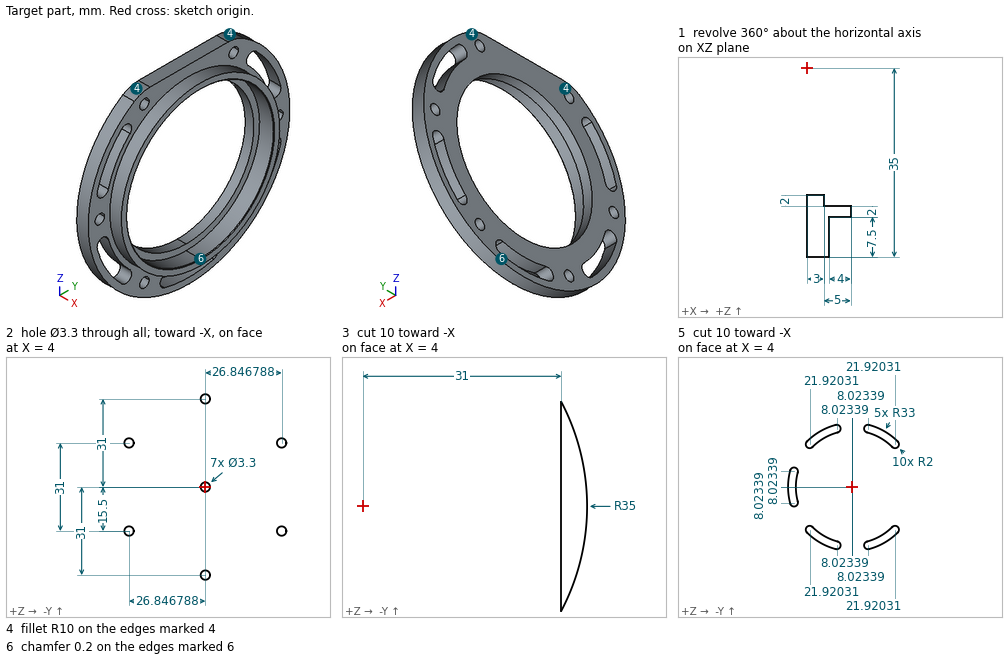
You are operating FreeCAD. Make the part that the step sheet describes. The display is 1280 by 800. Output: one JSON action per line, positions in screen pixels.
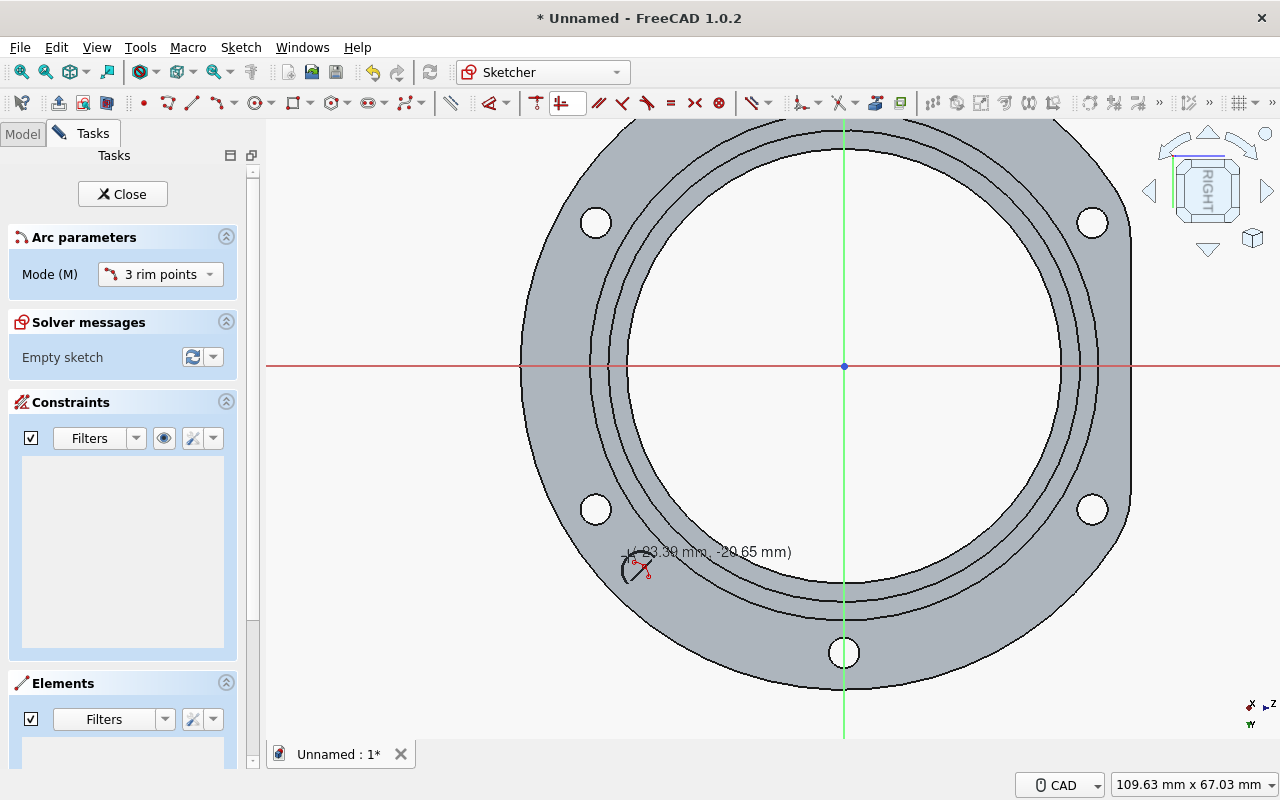
{"action": "left_click", "coordinate": [628, 556]}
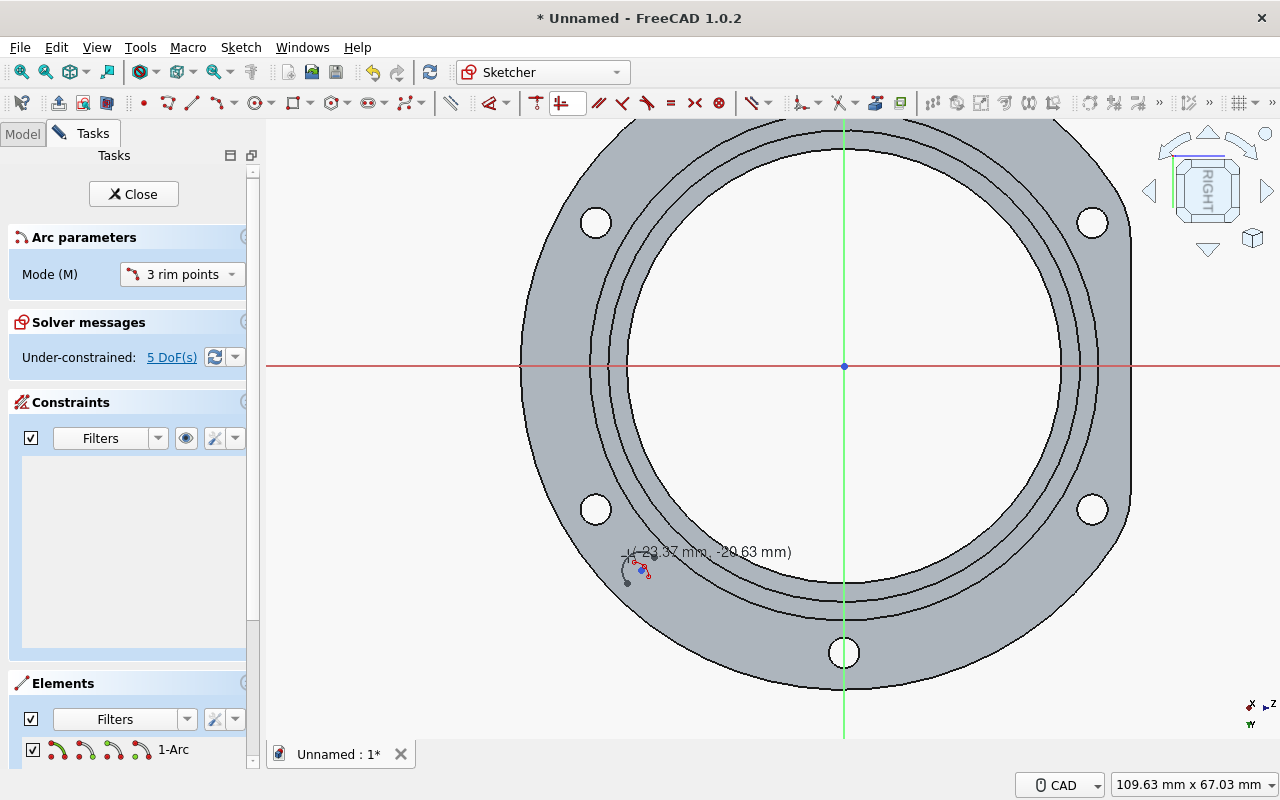
{"action": "left_click", "coordinate": [628, 584]}
{"action": "left_click", "coordinate": [765, 661]}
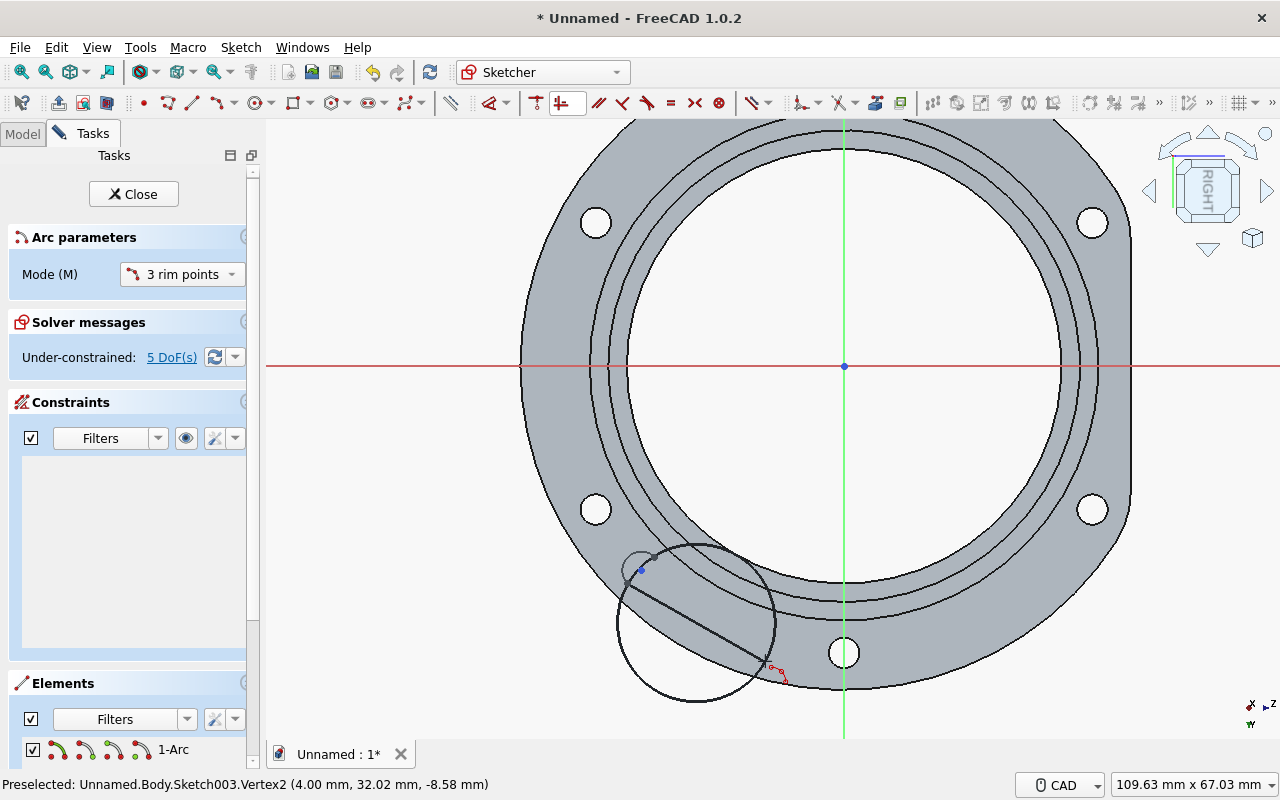
{"action": "scroll", "coordinate": [692, 631], "scroll_direction": "up", "scroll_amount": 3}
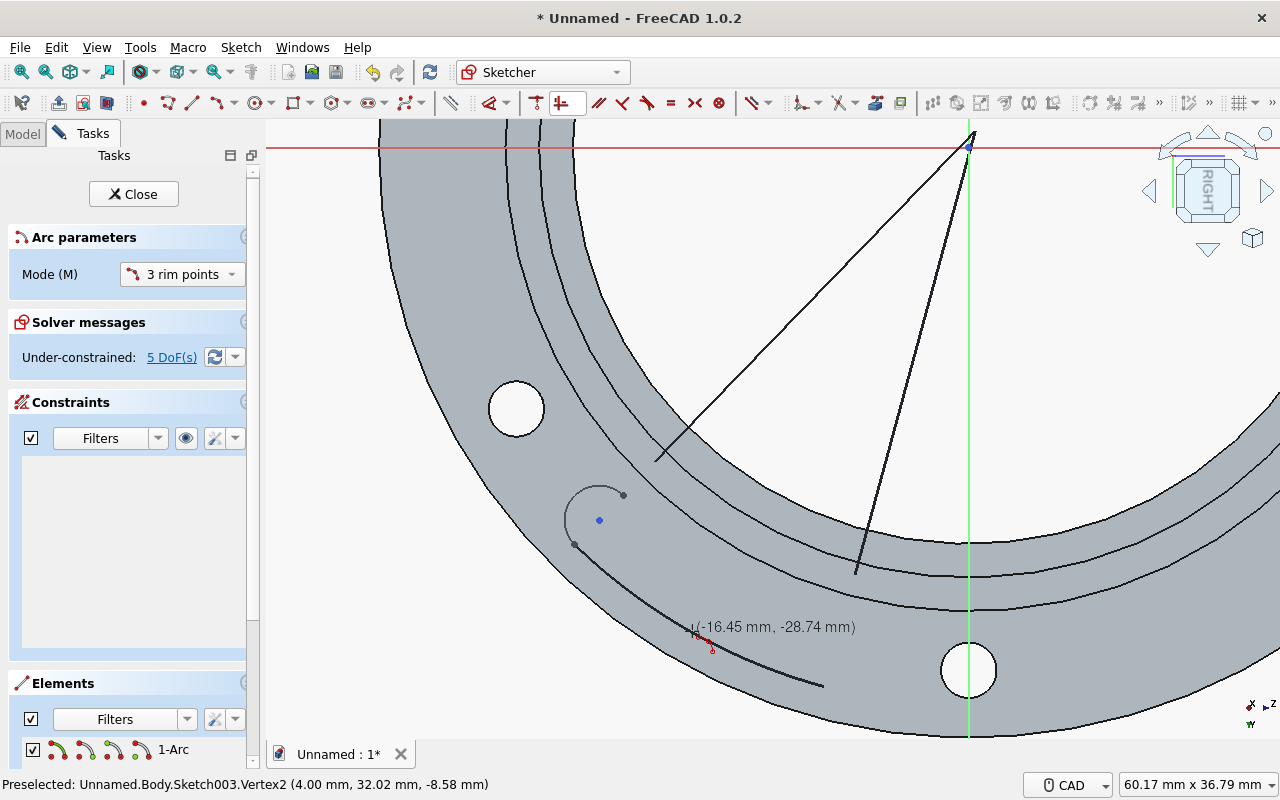
{"action": "left_click", "coordinate": [691, 629]}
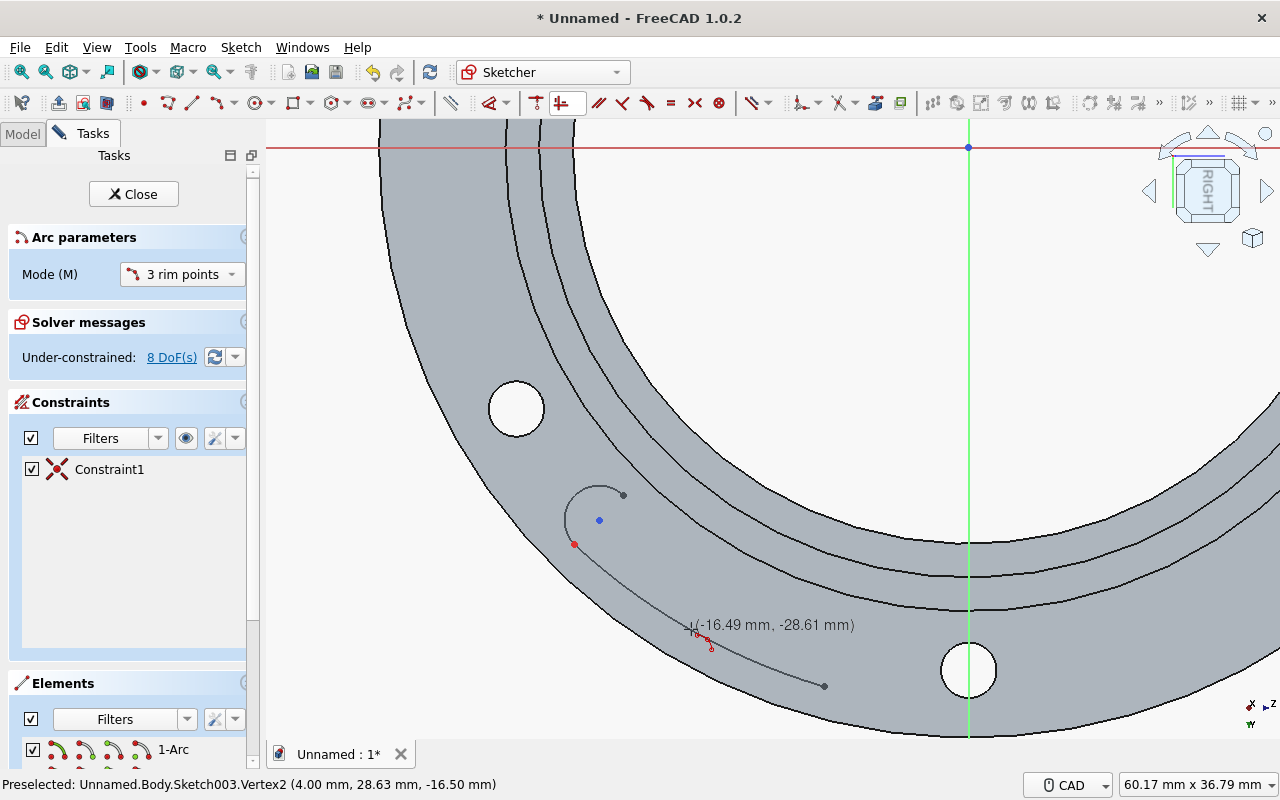
{"action": "left_click", "coordinate": [825, 687]}
{"action": "left_click", "coordinate": [842, 620]}
{"action": "left_click", "coordinate": [866, 661]}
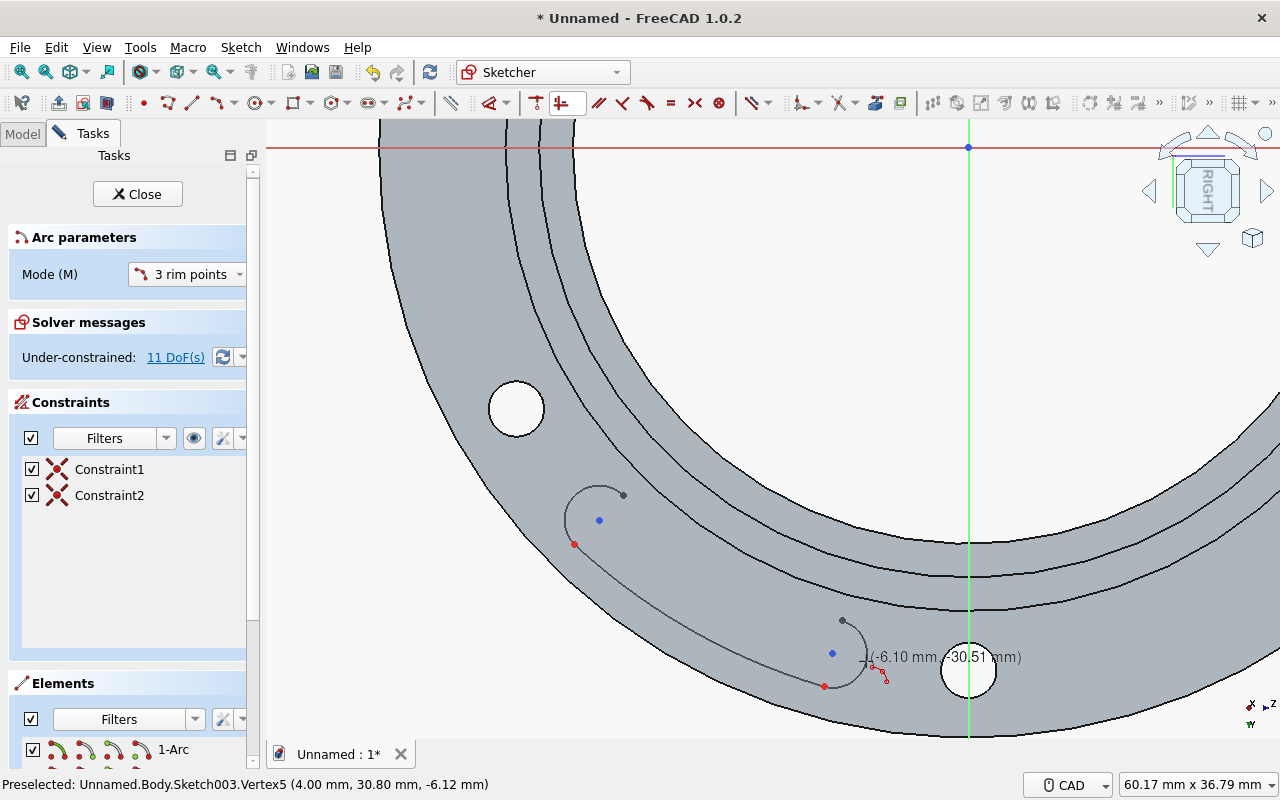
{"action": "left_click", "coordinate": [842, 621]}
{"action": "left_click", "coordinate": [624, 496]}
{"action": "left_click", "coordinate": [724, 571]}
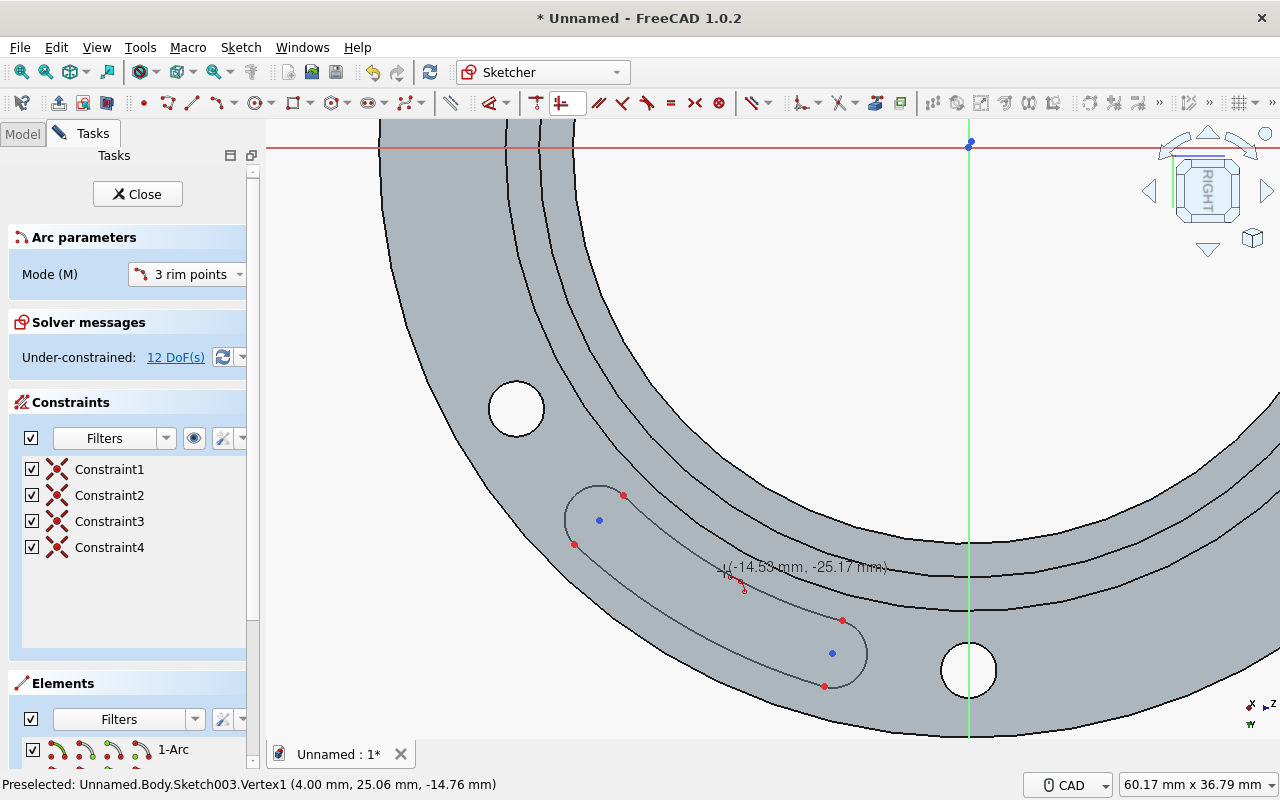
{"action": "left_click", "coordinate": [497, 274]}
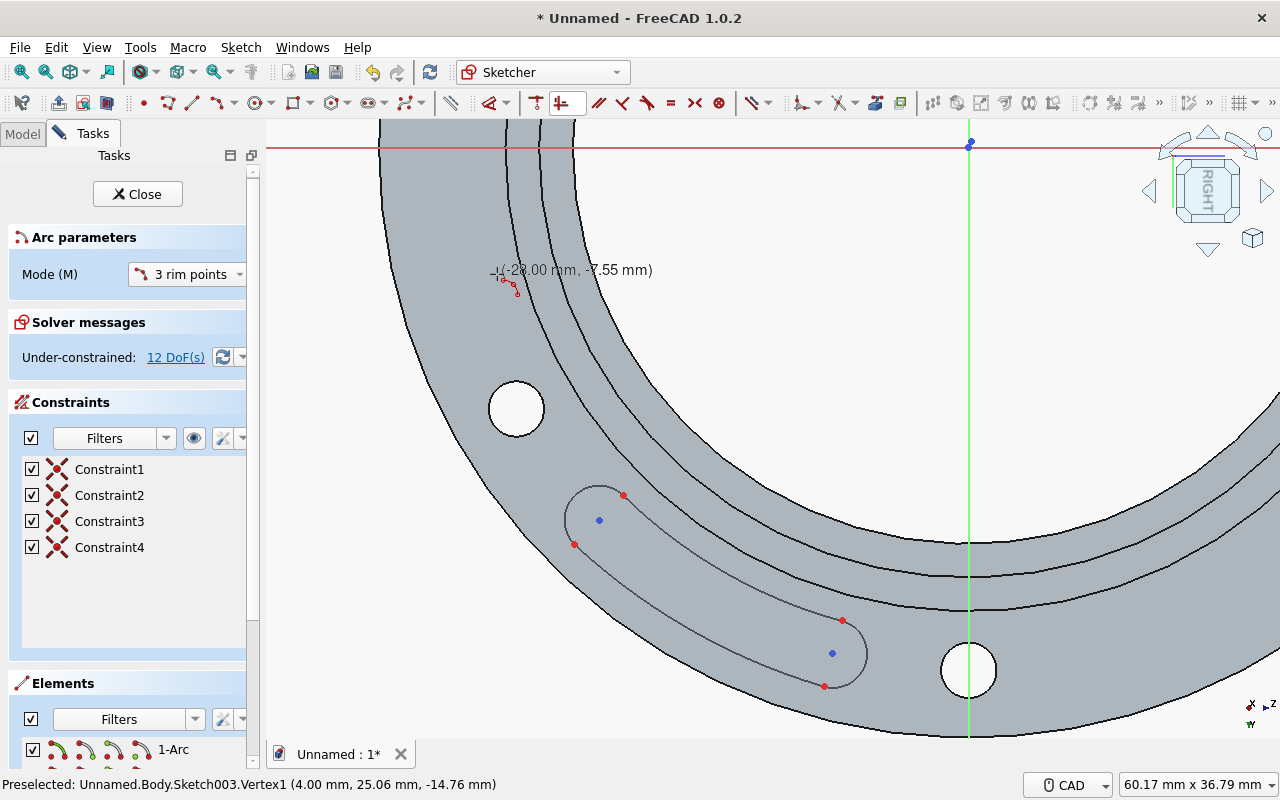
{"action": "scroll", "coordinate": [598, 593], "scroll_direction": "down", "scroll_amount": 5}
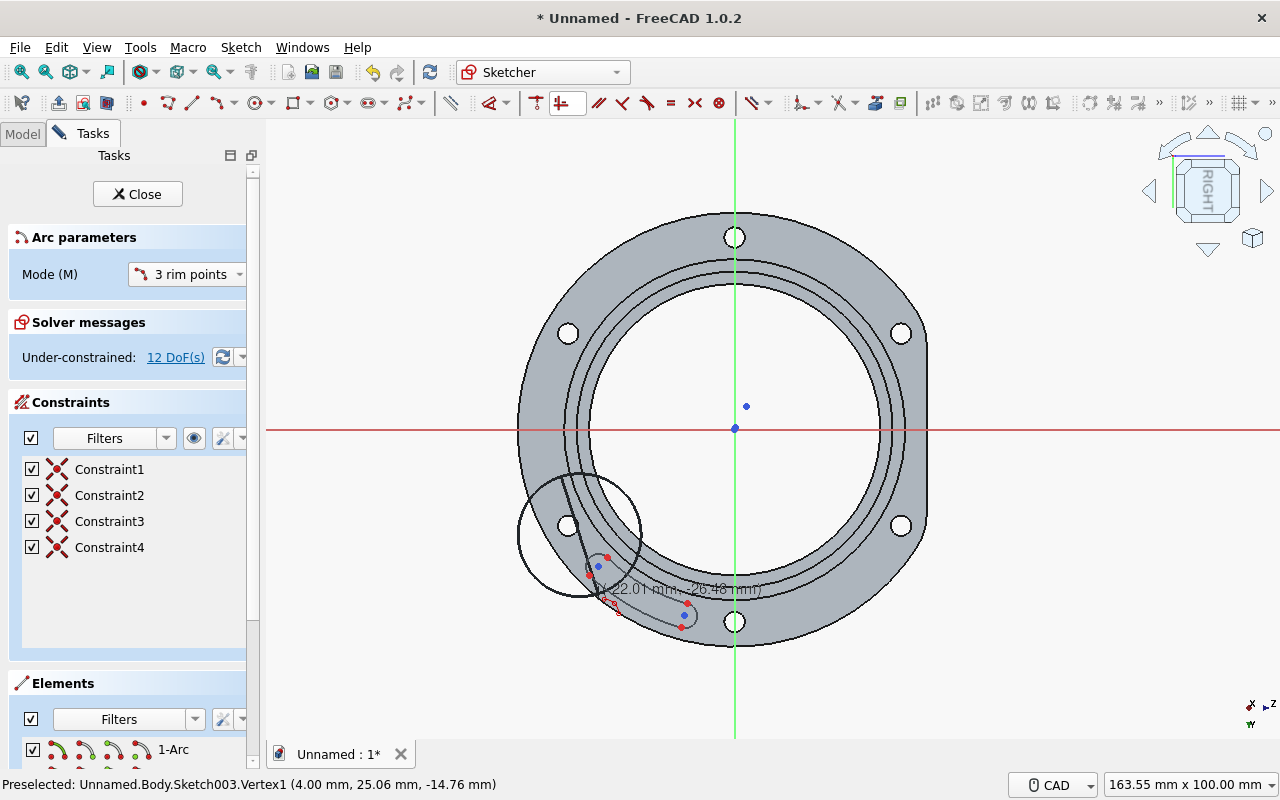
{"action": "left_click", "coordinate": [561, 383]}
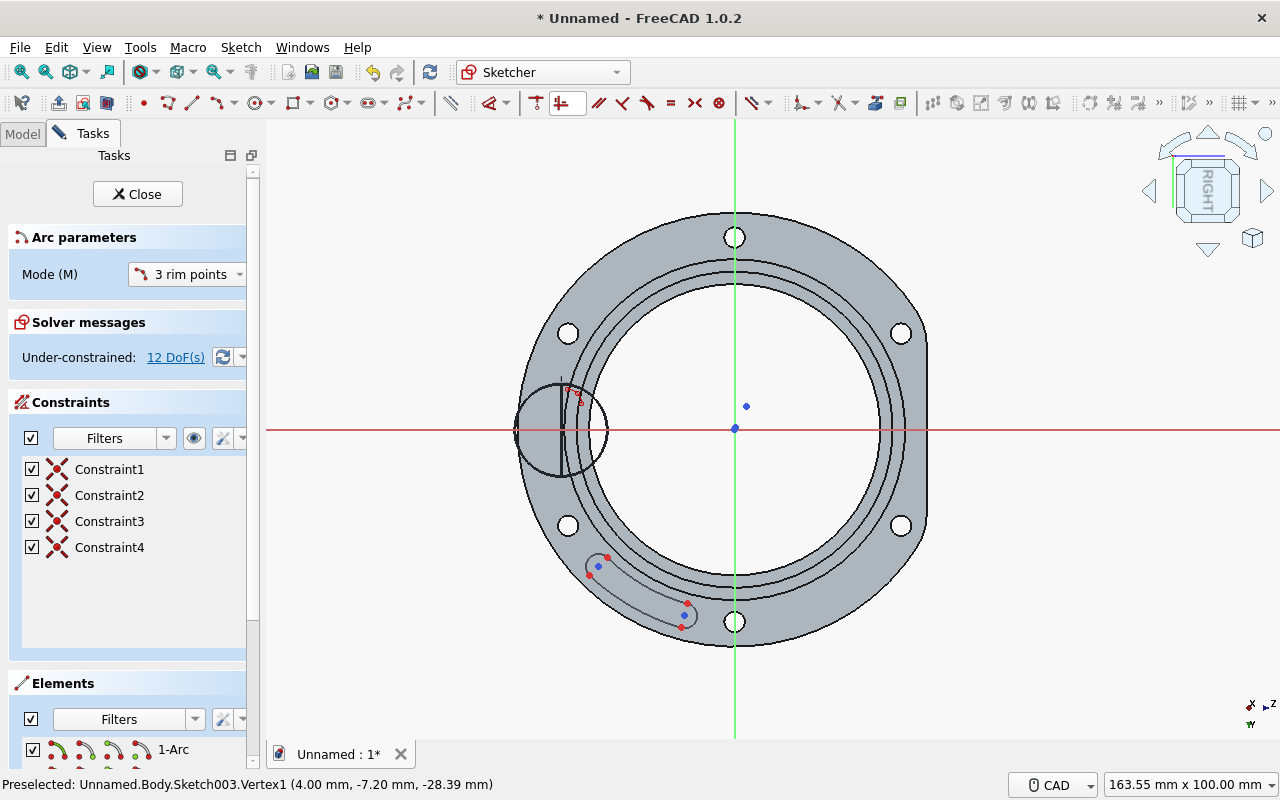
{"action": "scroll", "coordinate": [555, 420], "scroll_direction": "up", "scroll_amount": 5}